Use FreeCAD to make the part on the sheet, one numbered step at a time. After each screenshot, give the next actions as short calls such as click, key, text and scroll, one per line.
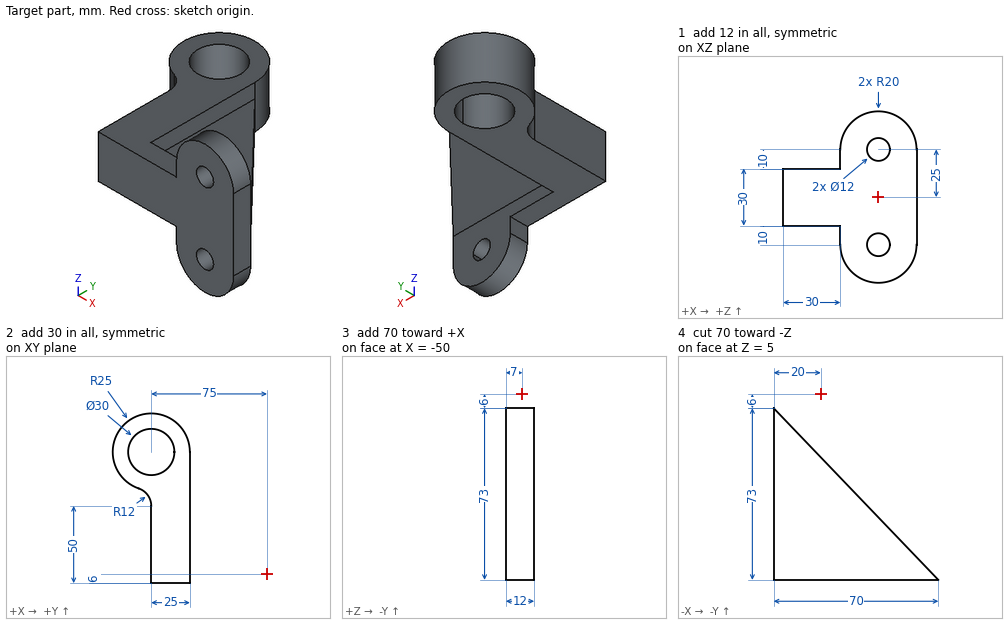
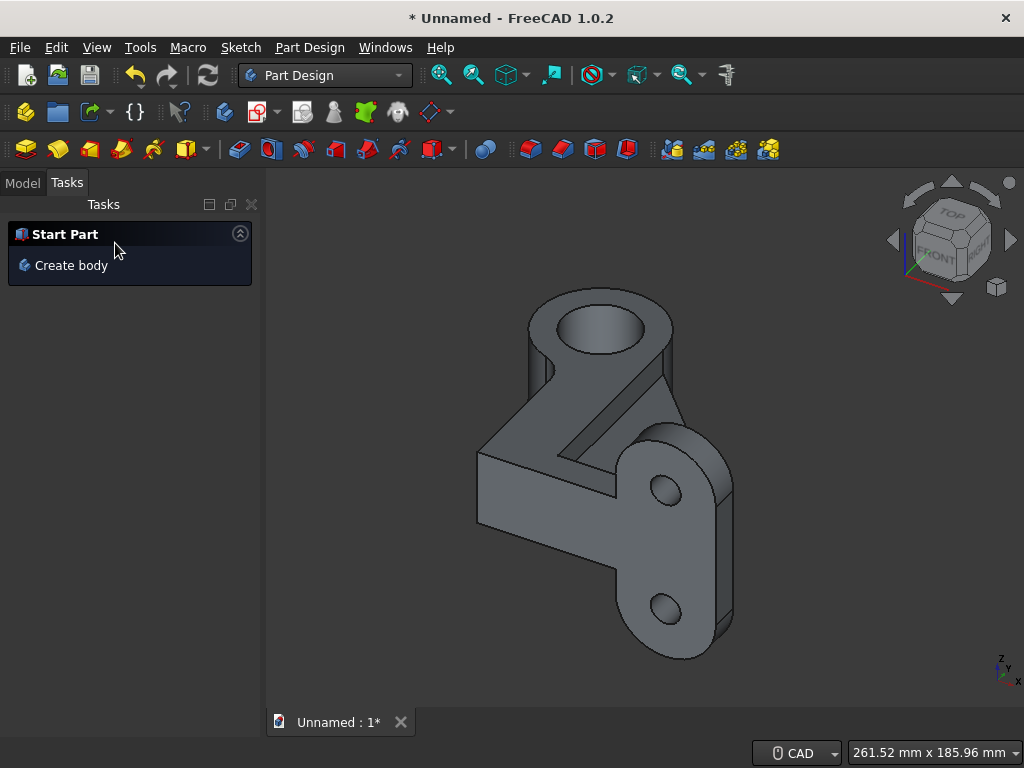
key(0)